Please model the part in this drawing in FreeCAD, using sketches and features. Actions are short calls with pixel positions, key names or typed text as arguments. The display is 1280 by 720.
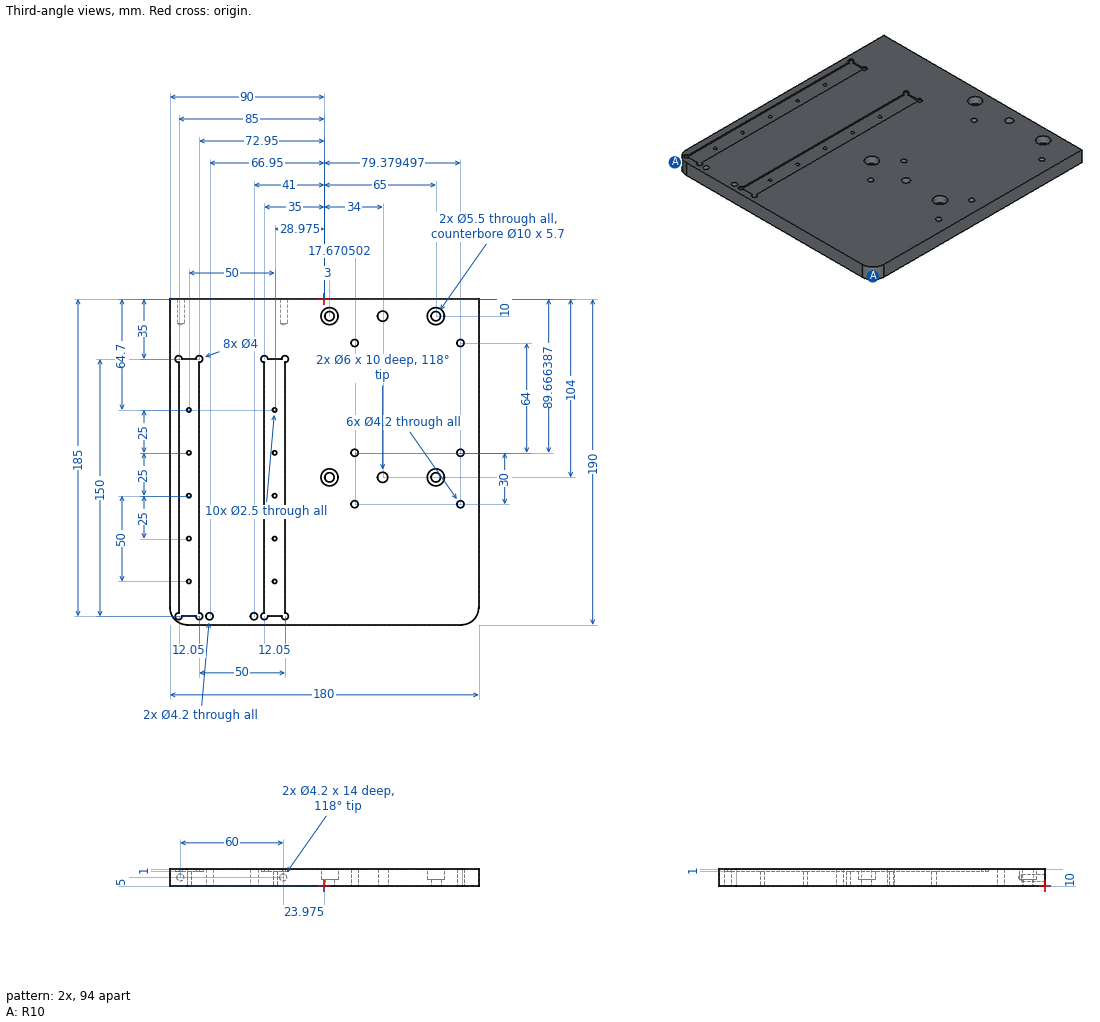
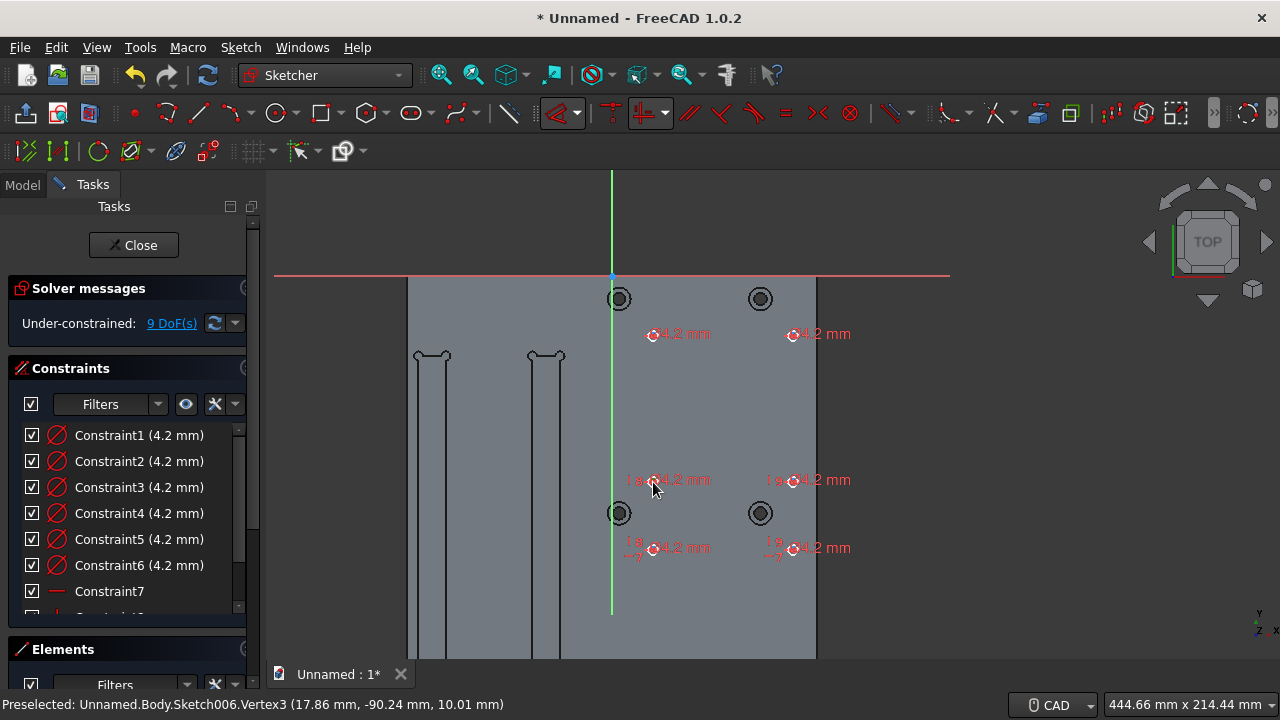
click(793, 482)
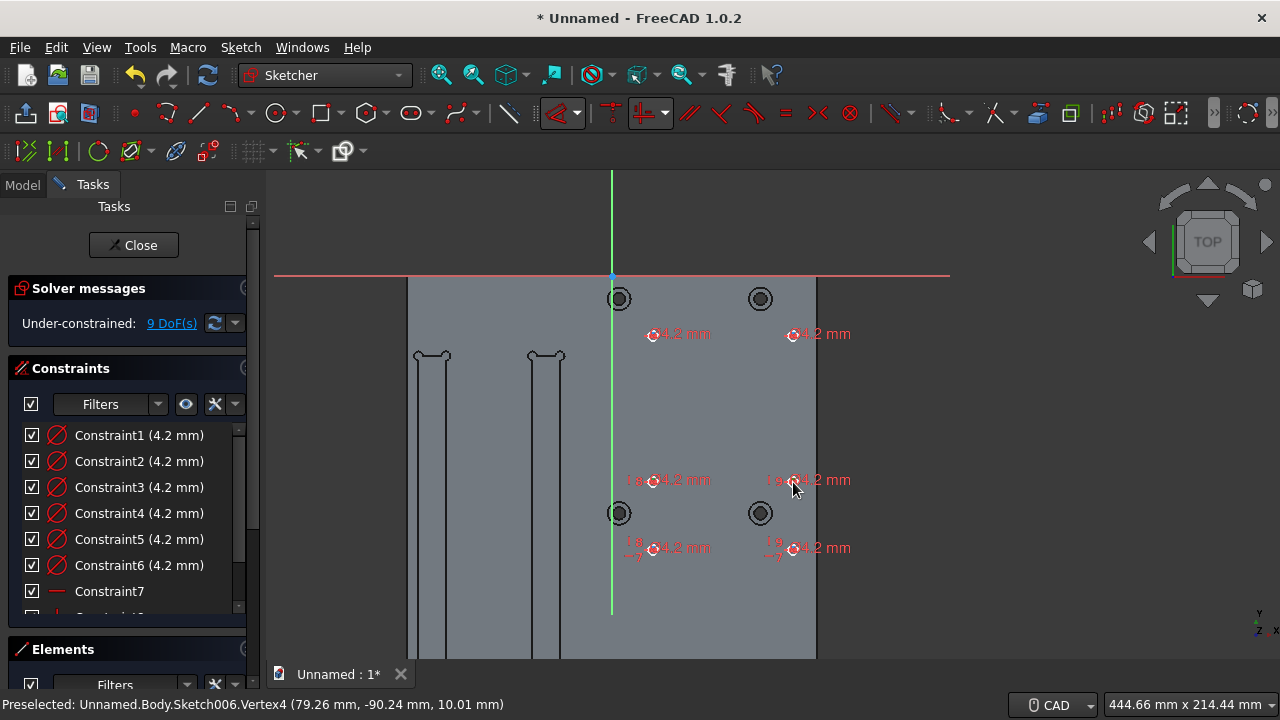
key(h)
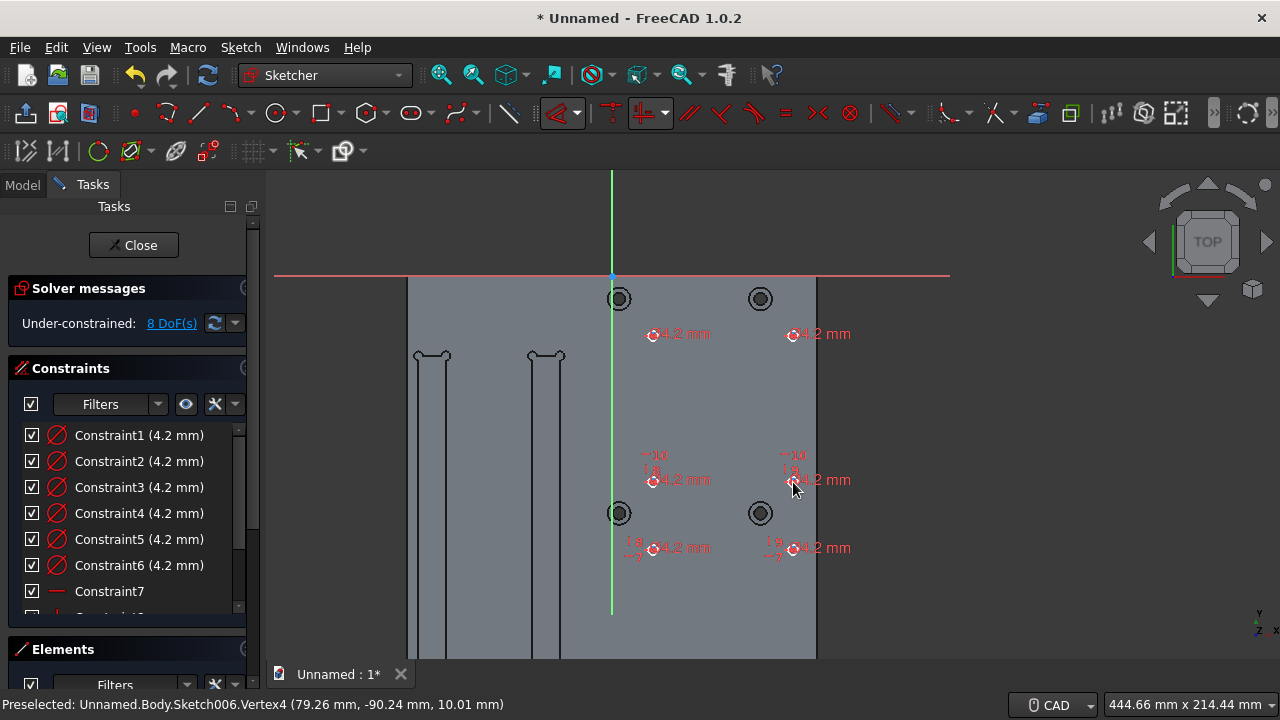
click(793, 482)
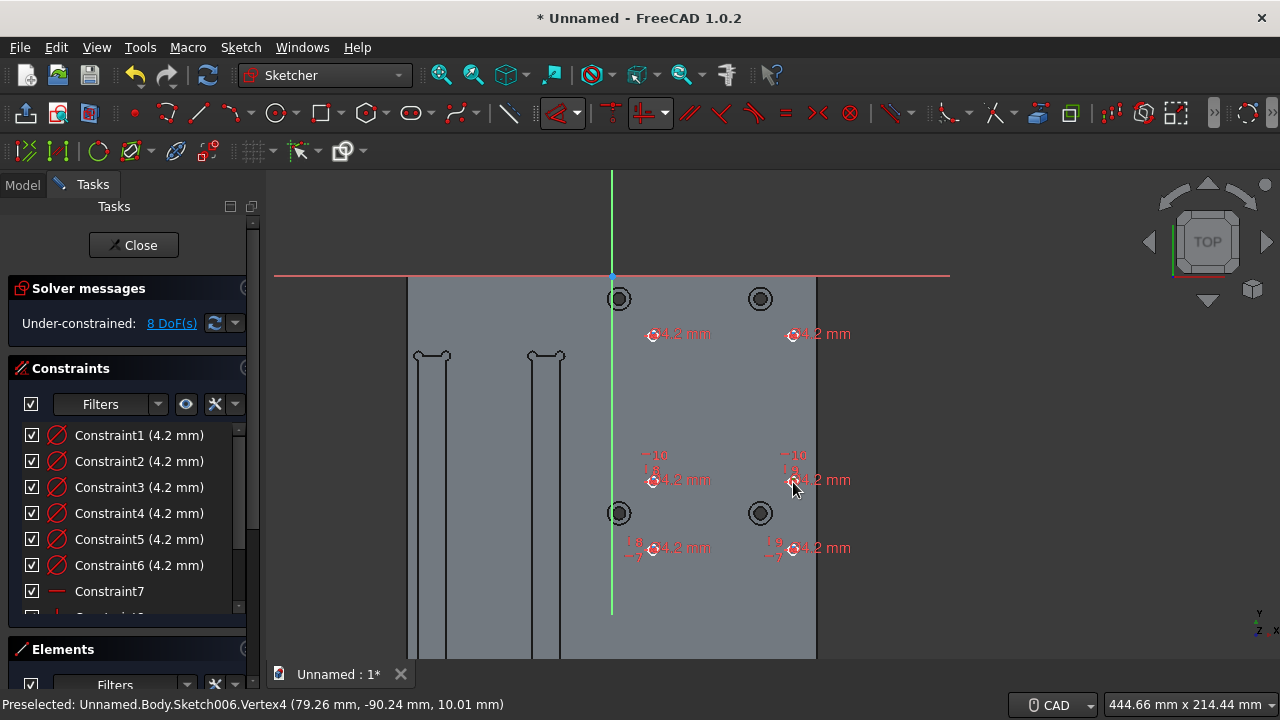
click(793, 336)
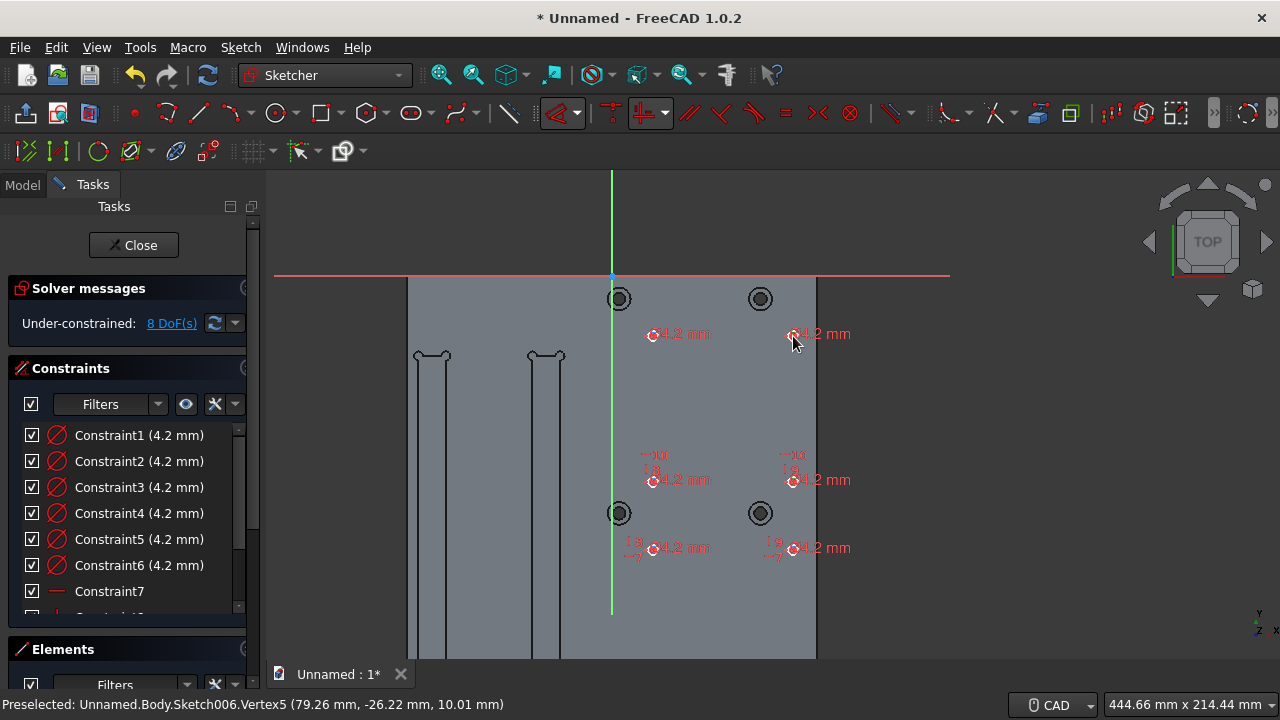
key(v)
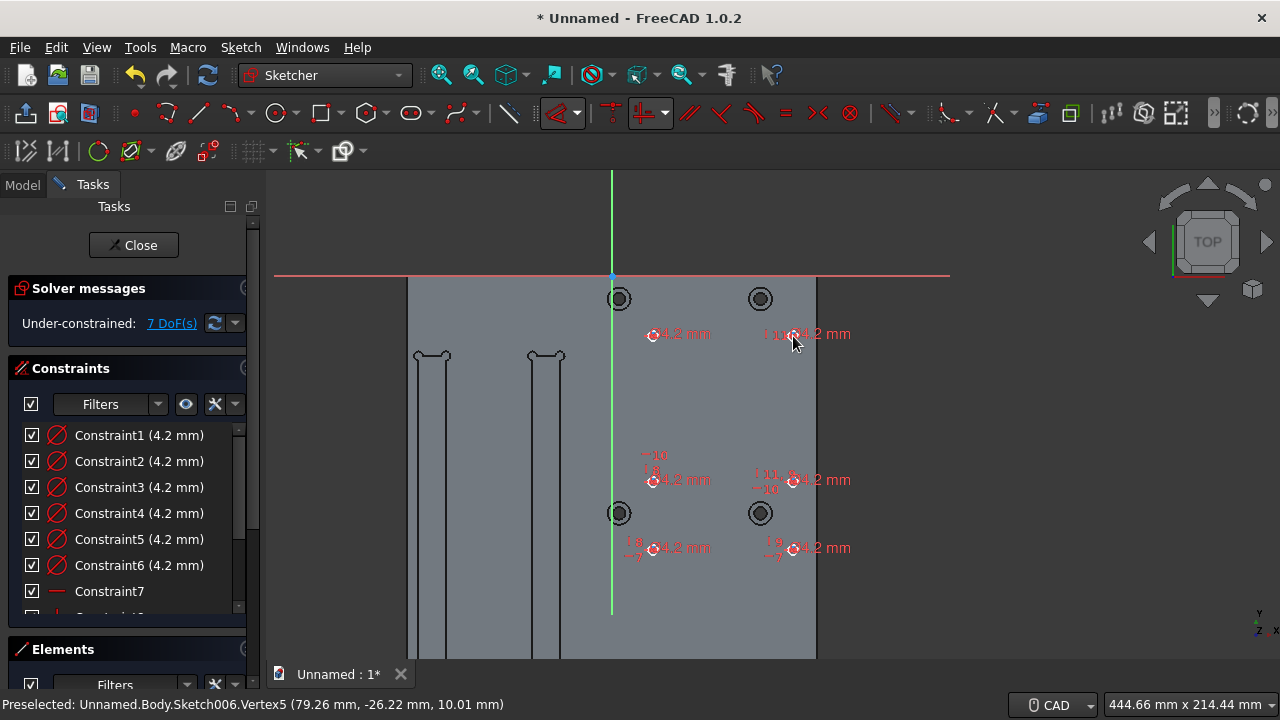
click(653, 482)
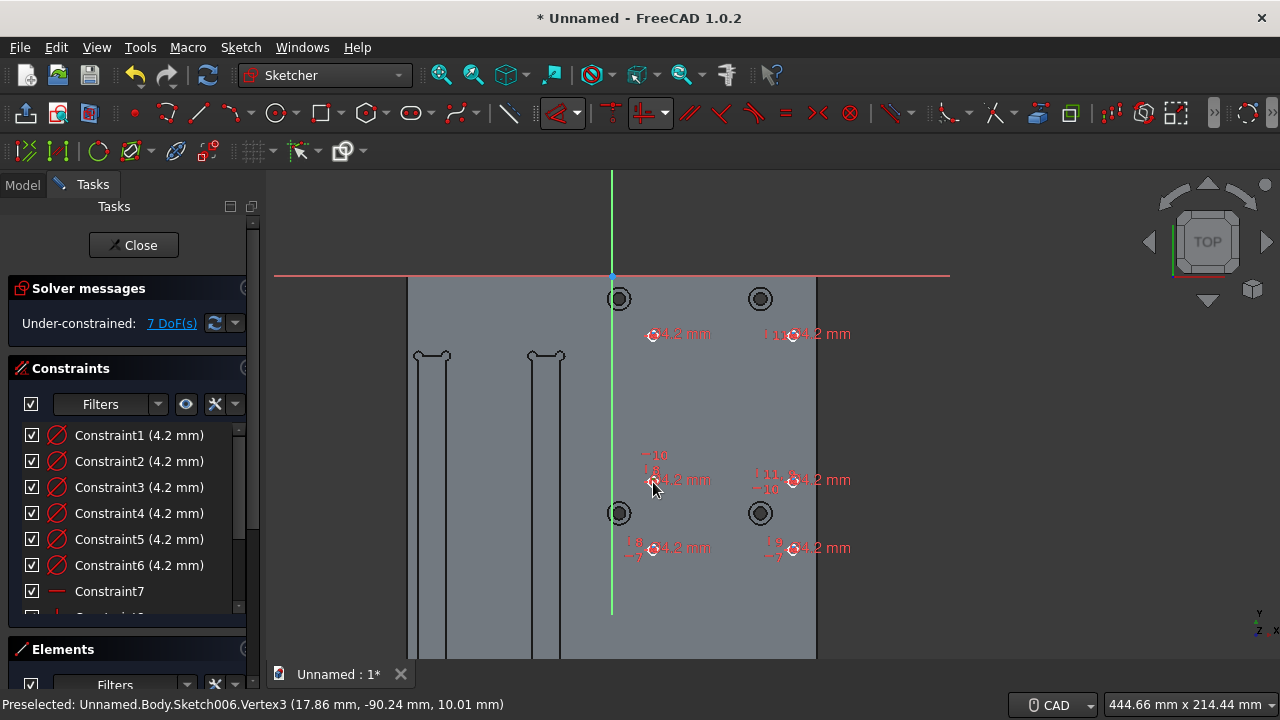
click(653, 336)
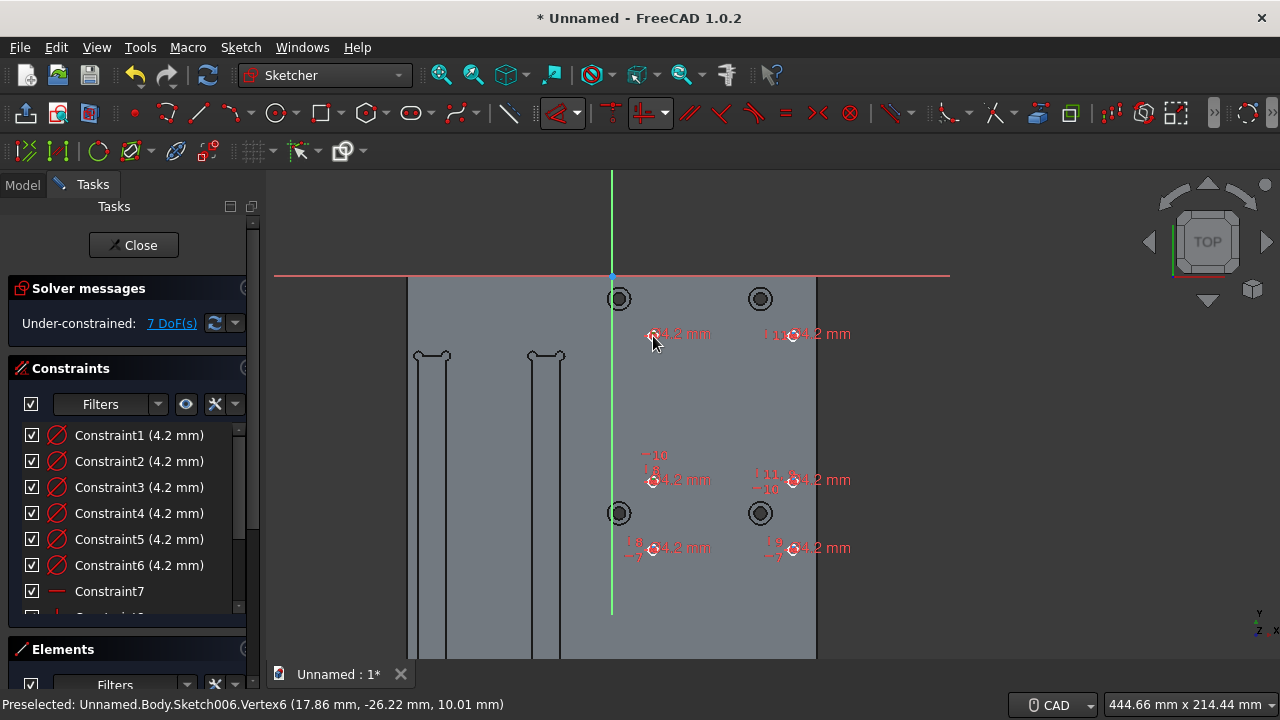
key(v)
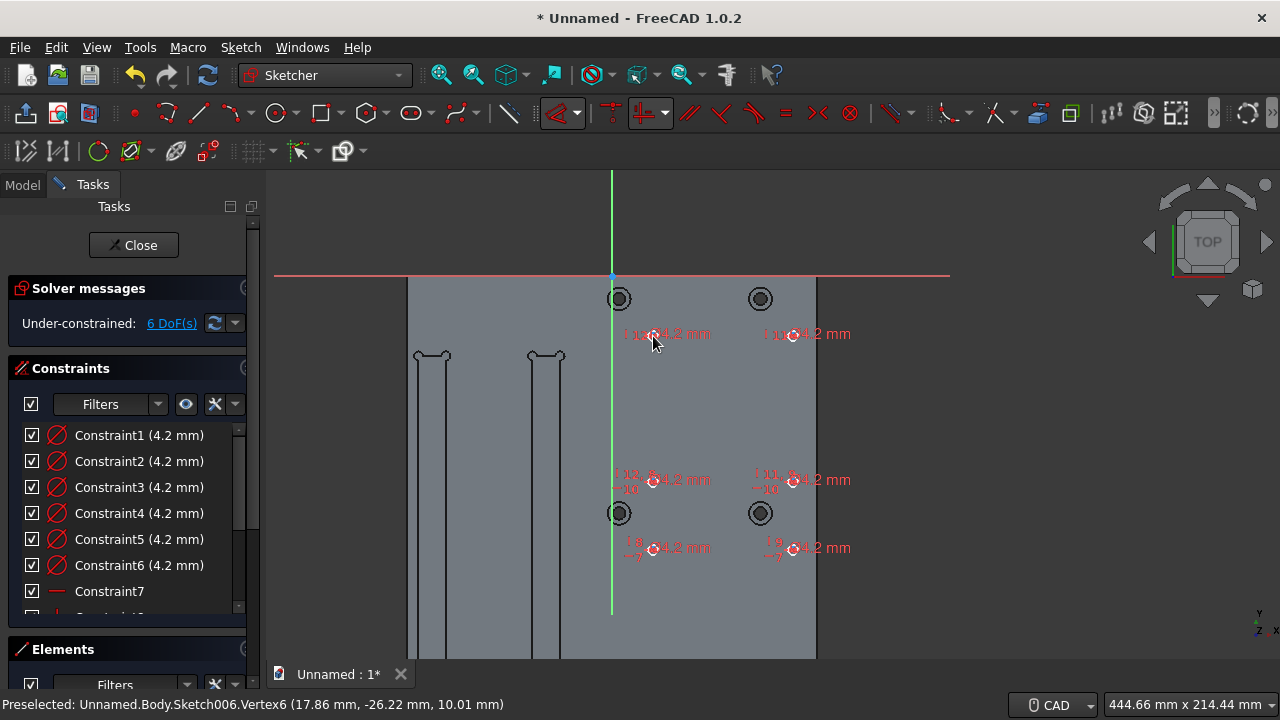
click(793, 336)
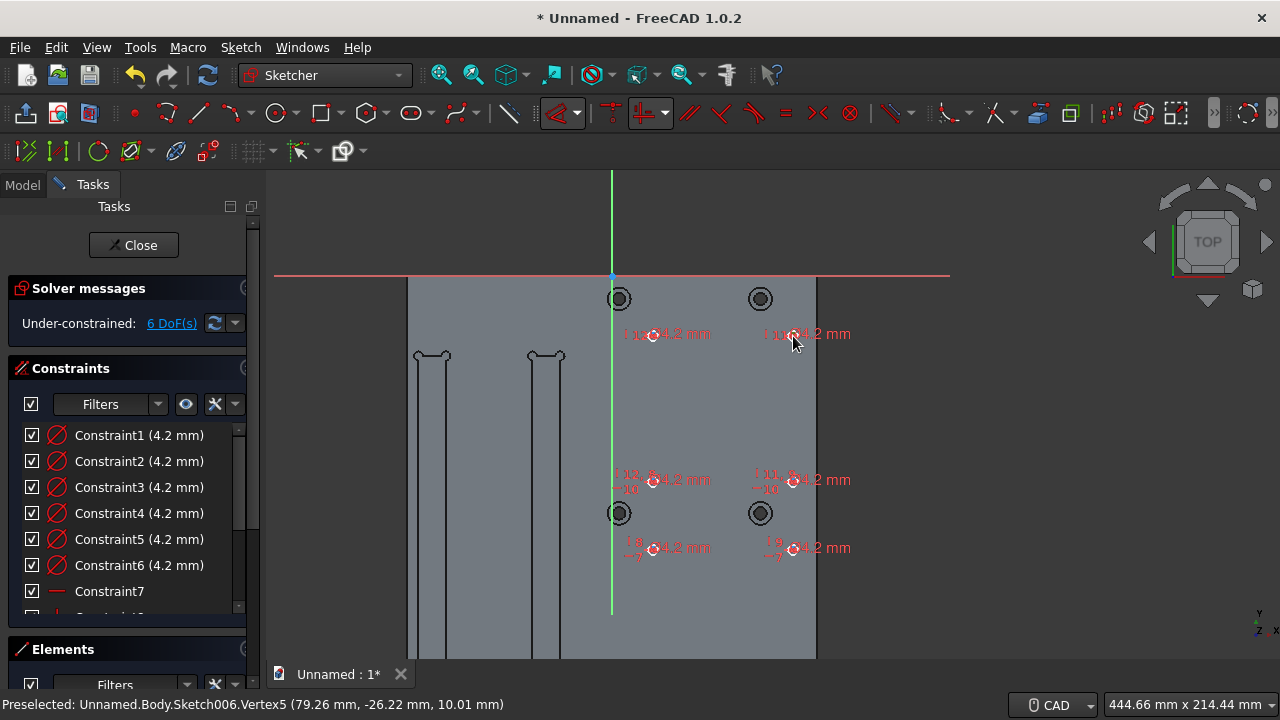
click(653, 336)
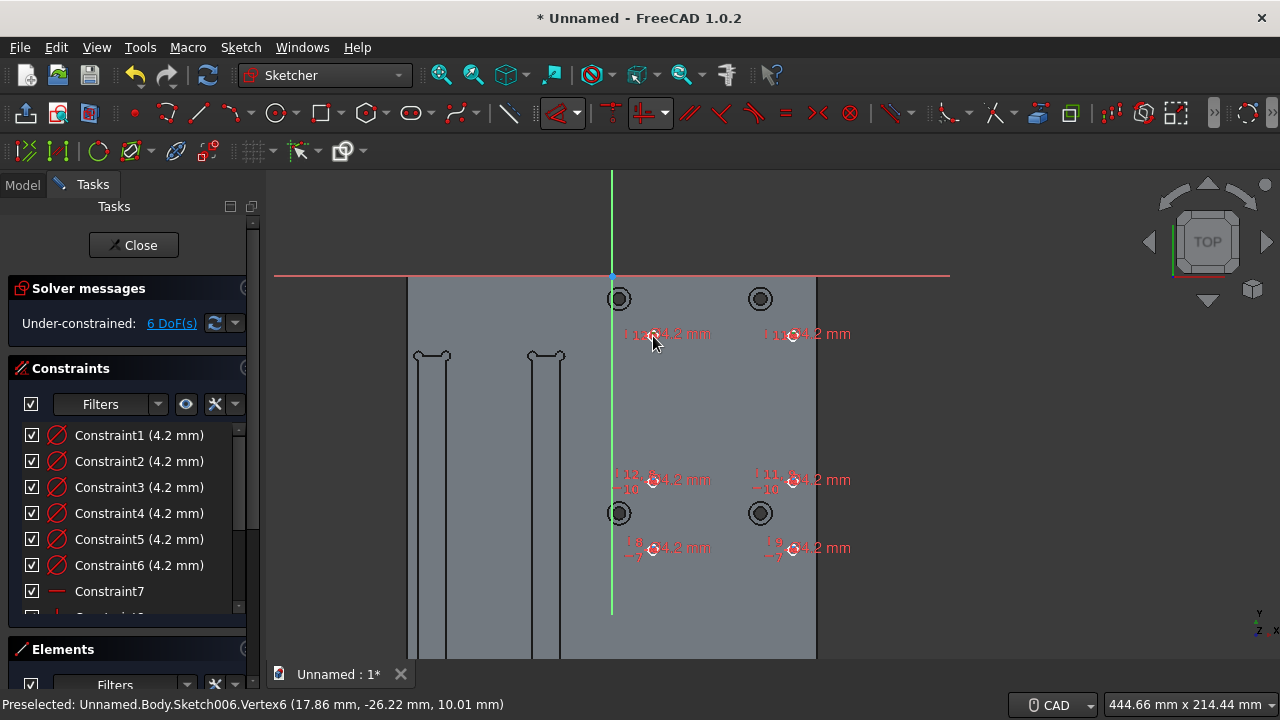
key(h)